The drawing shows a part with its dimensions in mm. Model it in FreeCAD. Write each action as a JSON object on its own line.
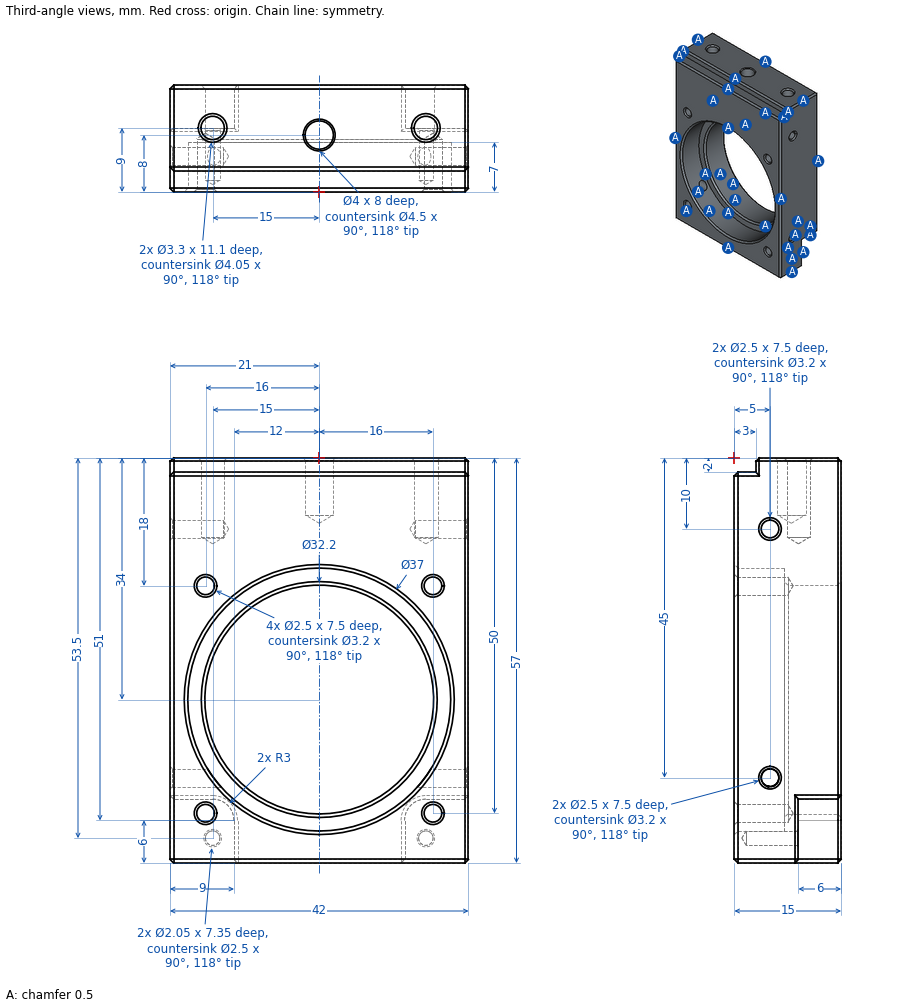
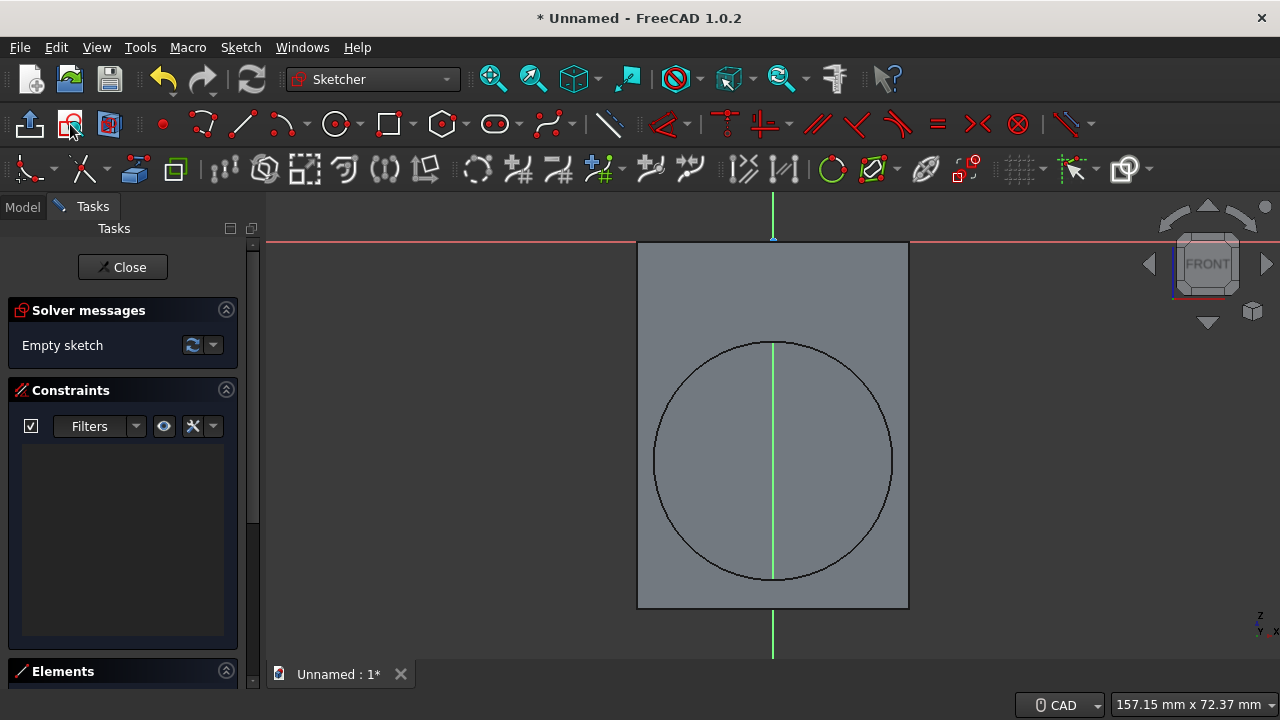
{"action": "scroll", "coordinate": [395, 526], "scroll_direction": "down", "scroll_amount": 1}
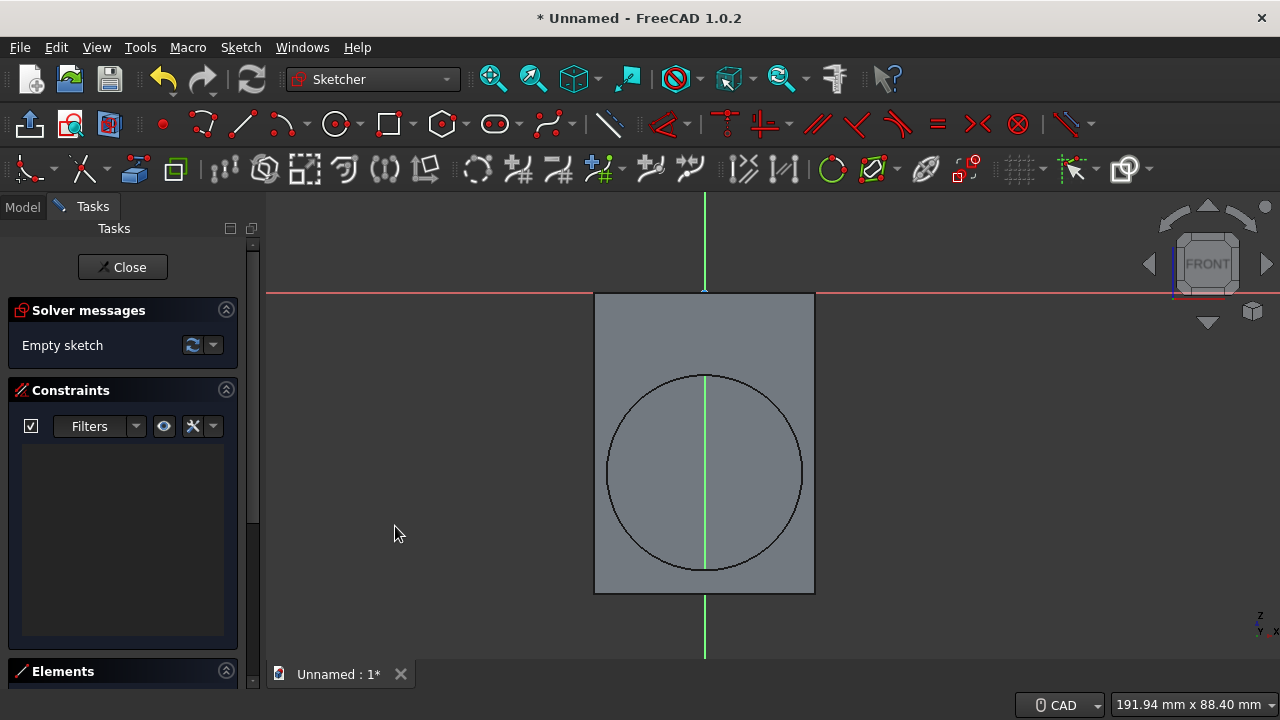
{"action": "left_click", "coordinate": [336, 124]}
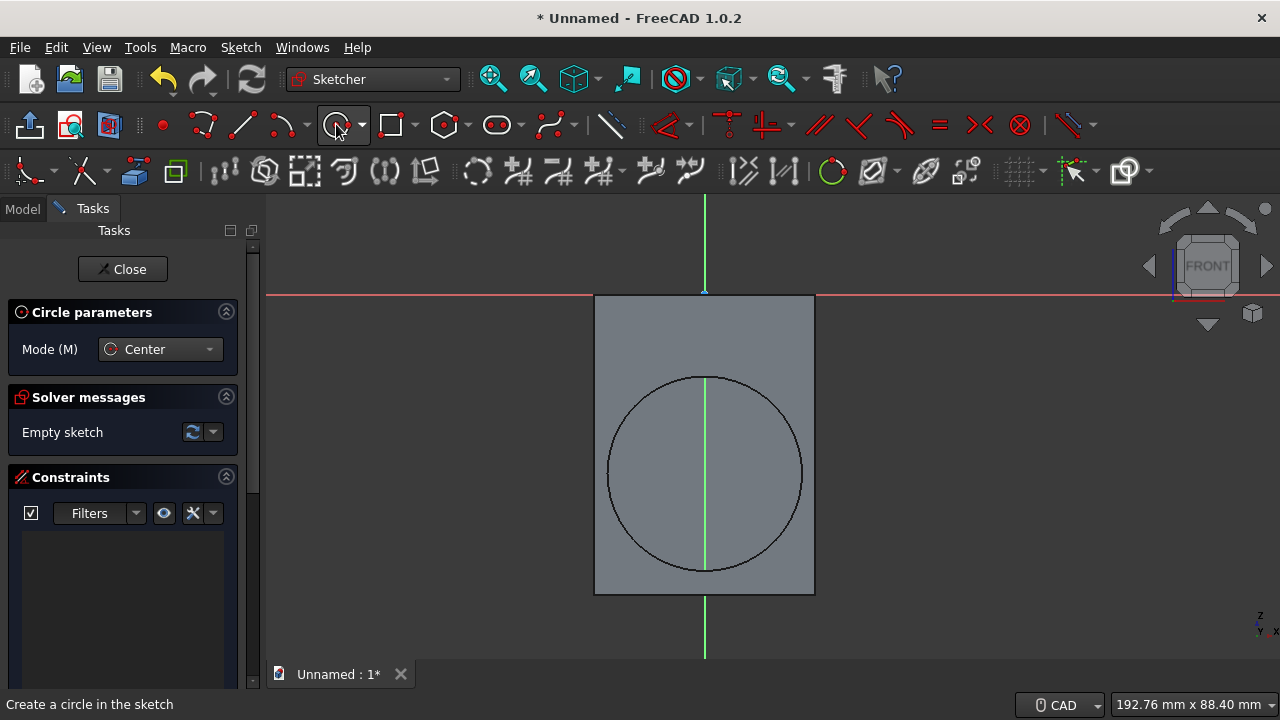
{"action": "left_click", "coordinate": [705, 474]}
{"action": "mouse_move", "coordinate": [765, 414]}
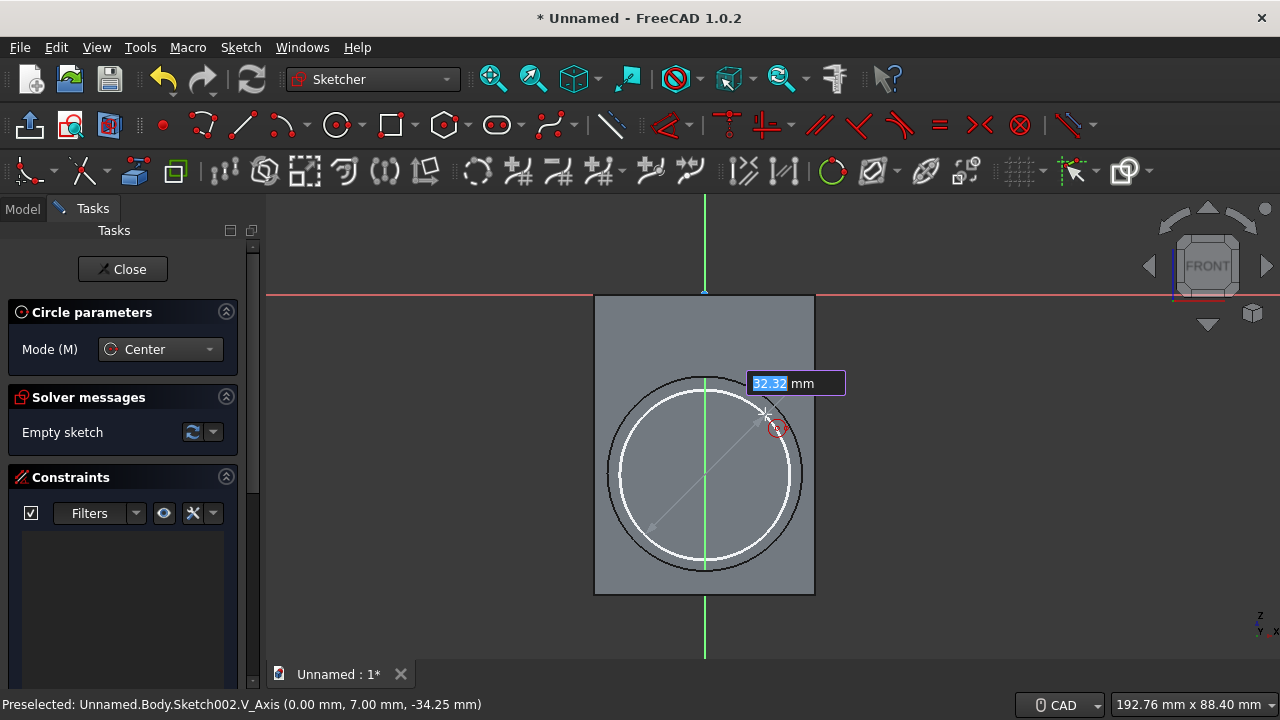
{"action": "type", "text": "32.2"}
{"action": "key", "text": "Return"}
{"action": "key", "text": "Escape"}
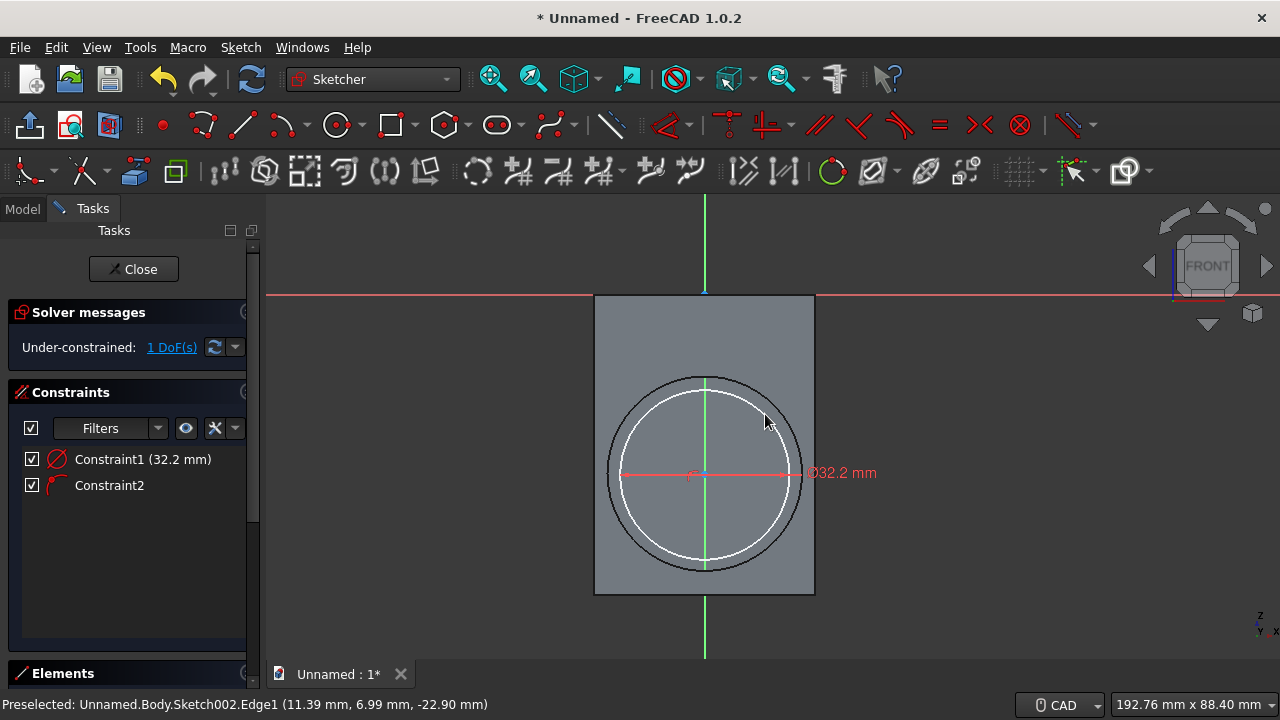
{"action": "key", "text": "d"}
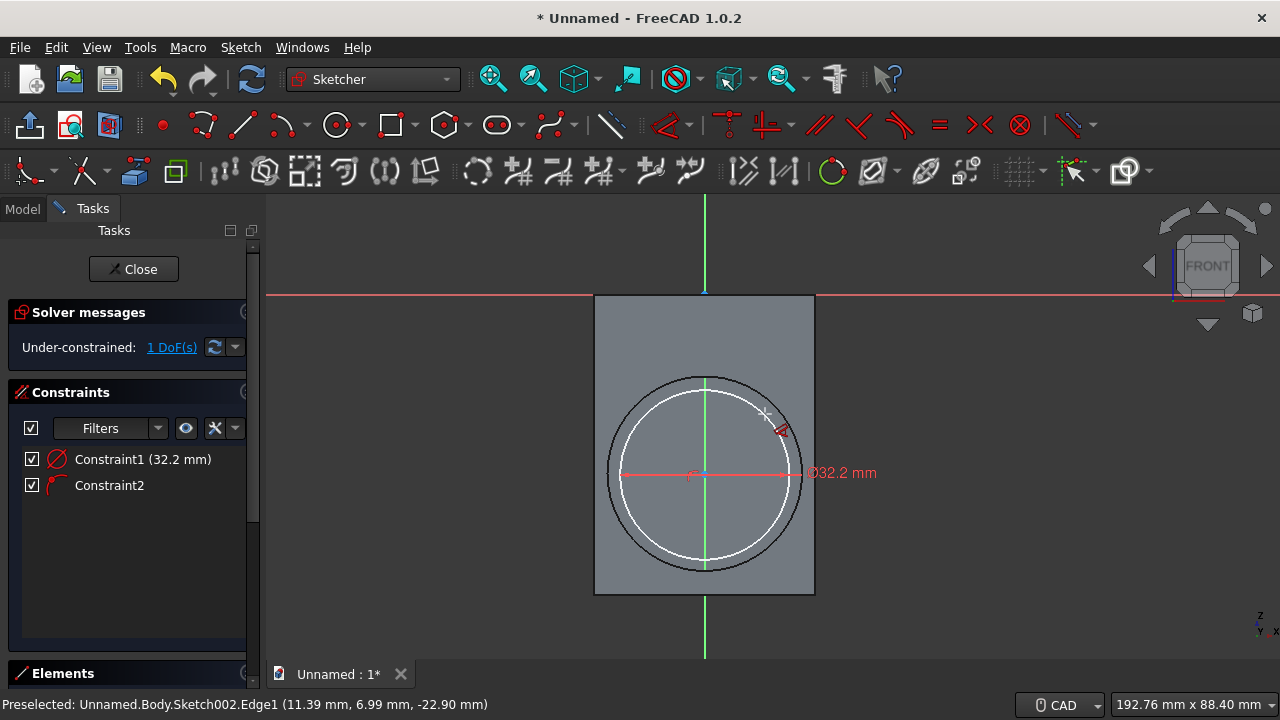
{"action": "left_click", "coordinate": [705, 475]}
{"action": "left_click", "coordinate": [739, 343]}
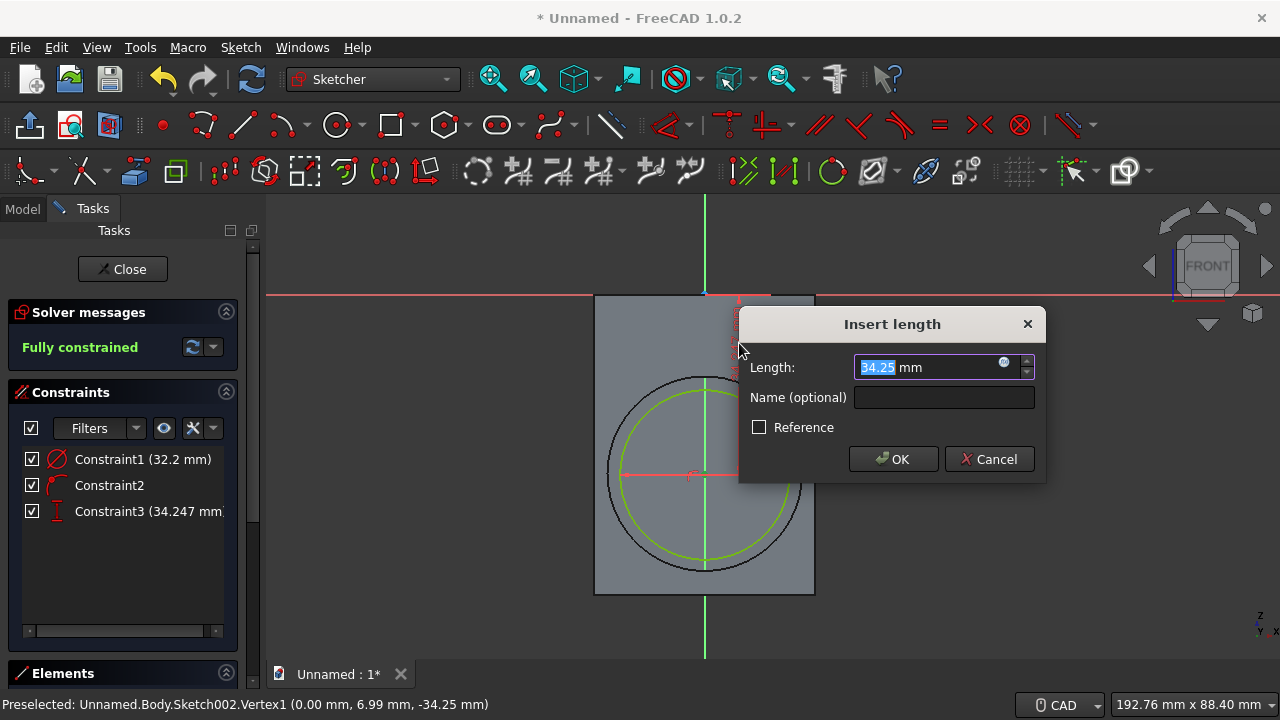
{"action": "type", "text": "34"}
{"action": "key", "text": "Return"}
{"action": "key", "text": "Escape"}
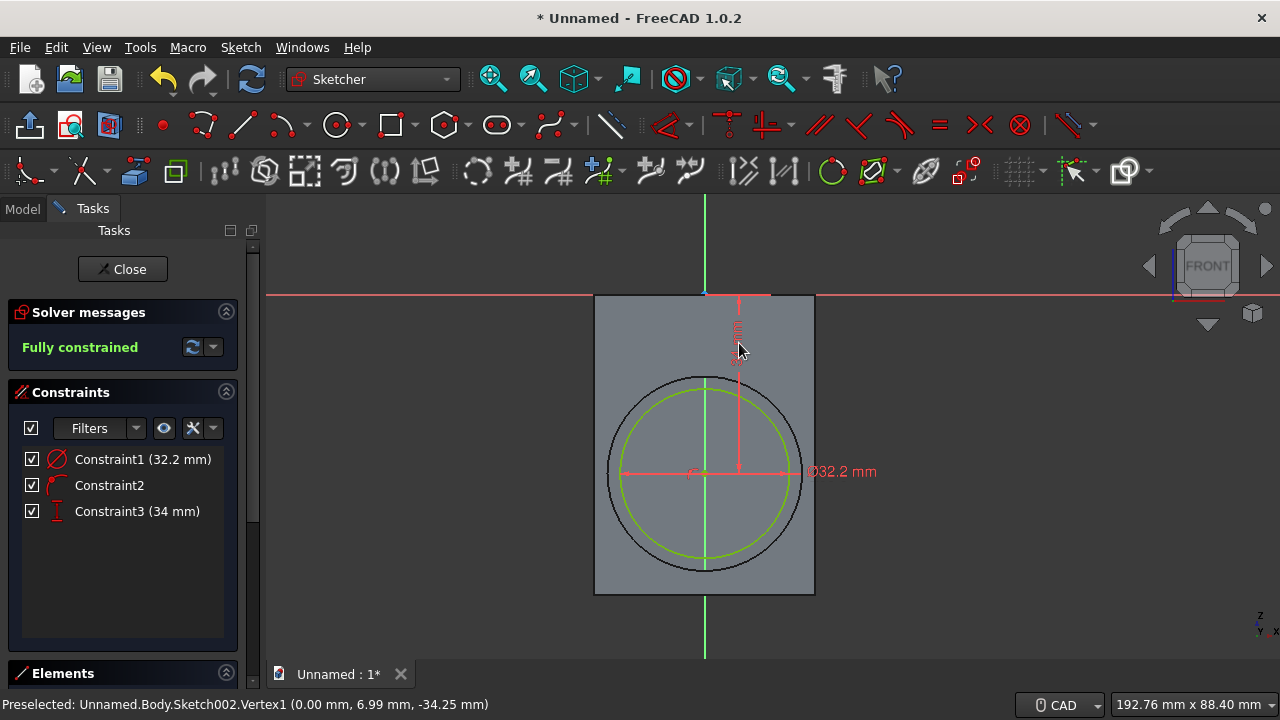
{"action": "left_click", "coordinate": [123, 269]}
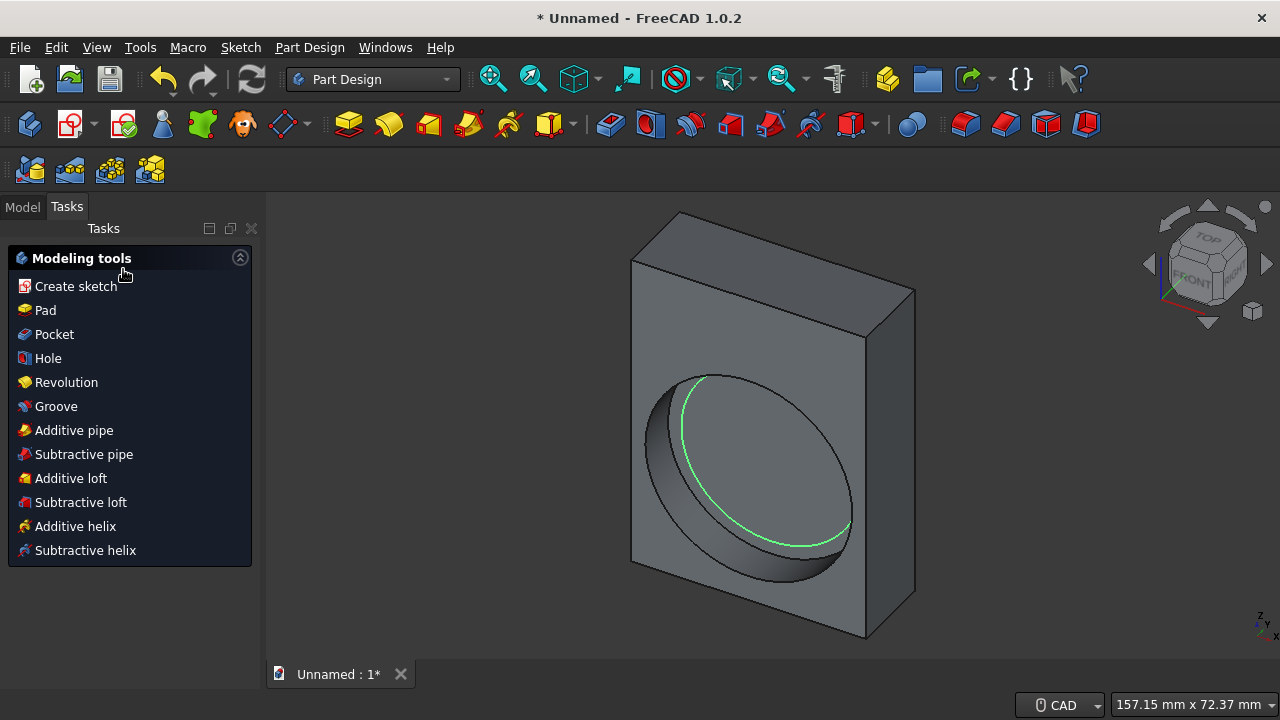
{"action": "left_click", "coordinate": [612, 124]}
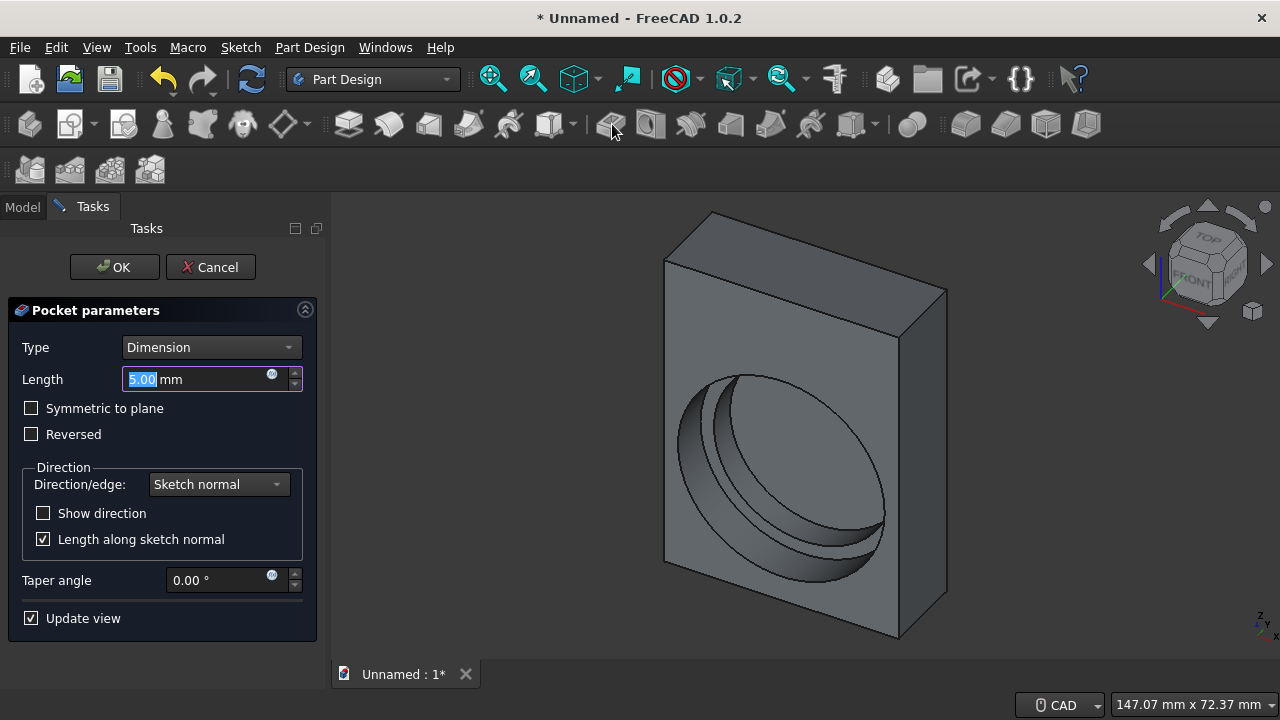
{"action": "left_click", "coordinate": [212, 348]}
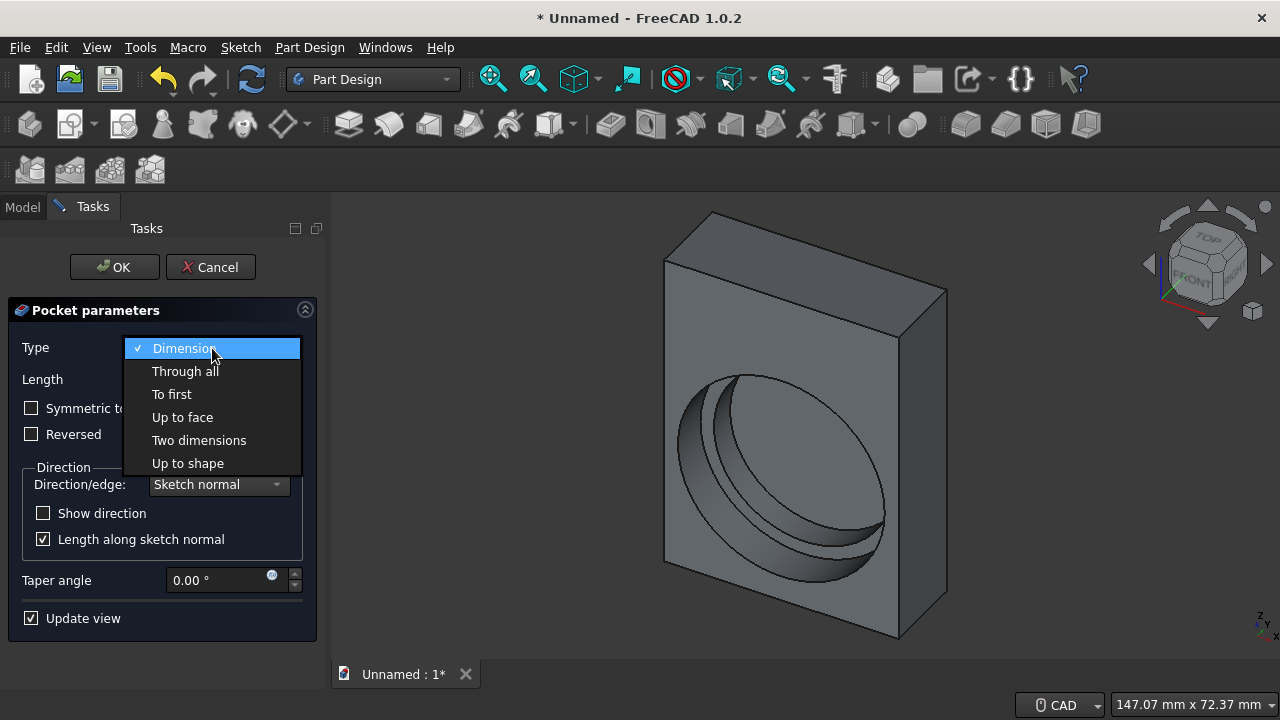
{"action": "left_click", "coordinate": [212, 372]}